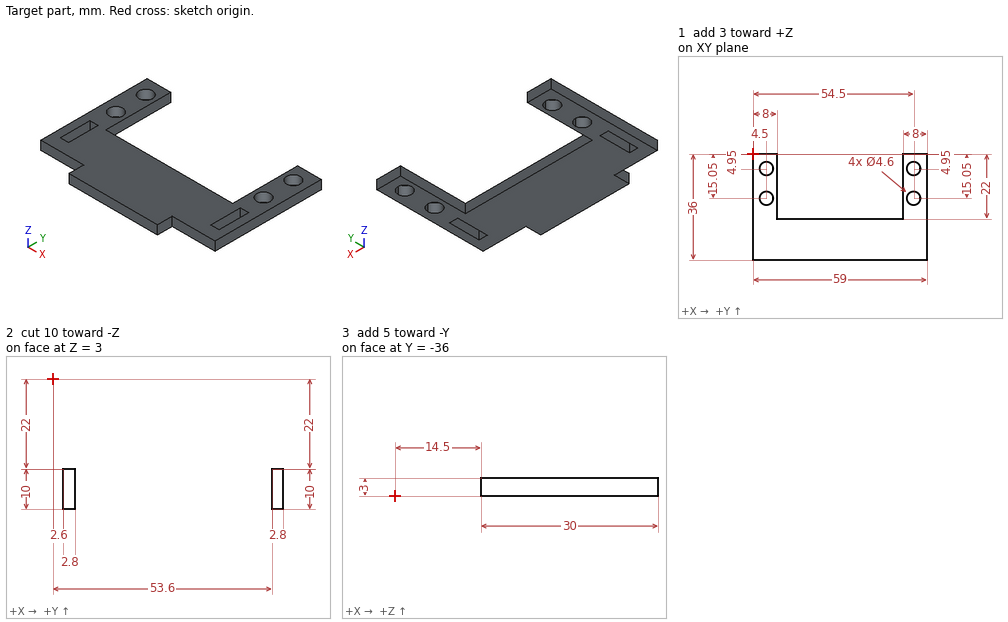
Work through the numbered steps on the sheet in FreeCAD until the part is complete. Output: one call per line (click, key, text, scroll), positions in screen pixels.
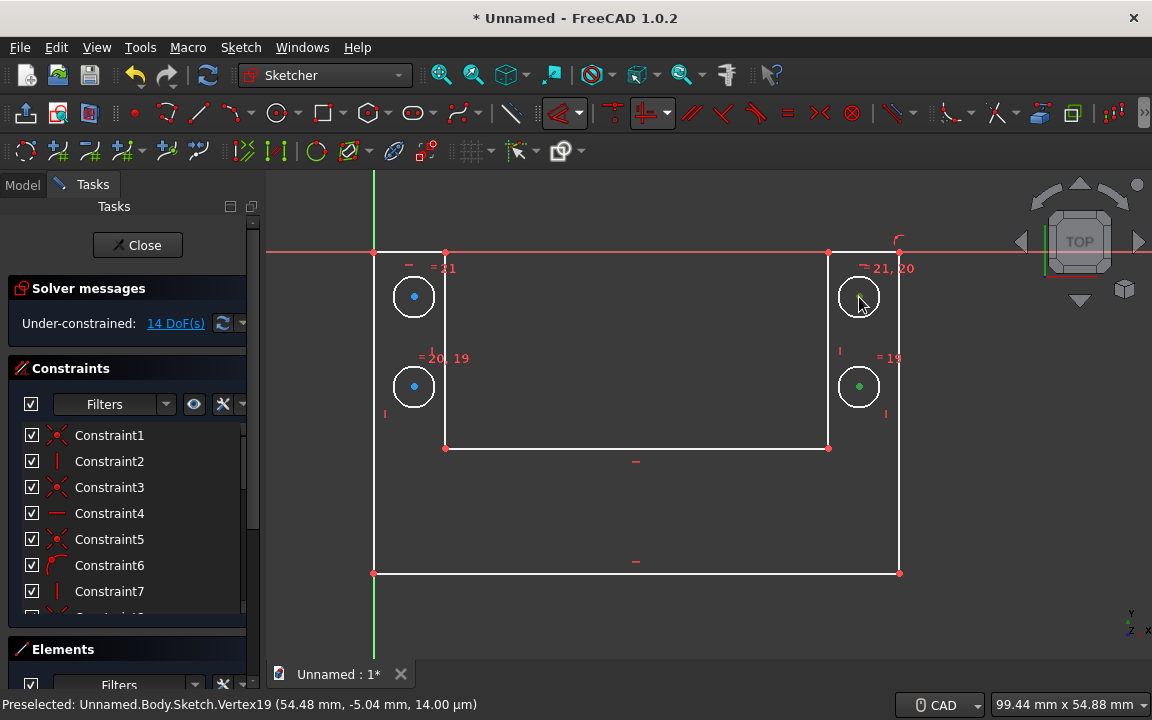
click(670, 114)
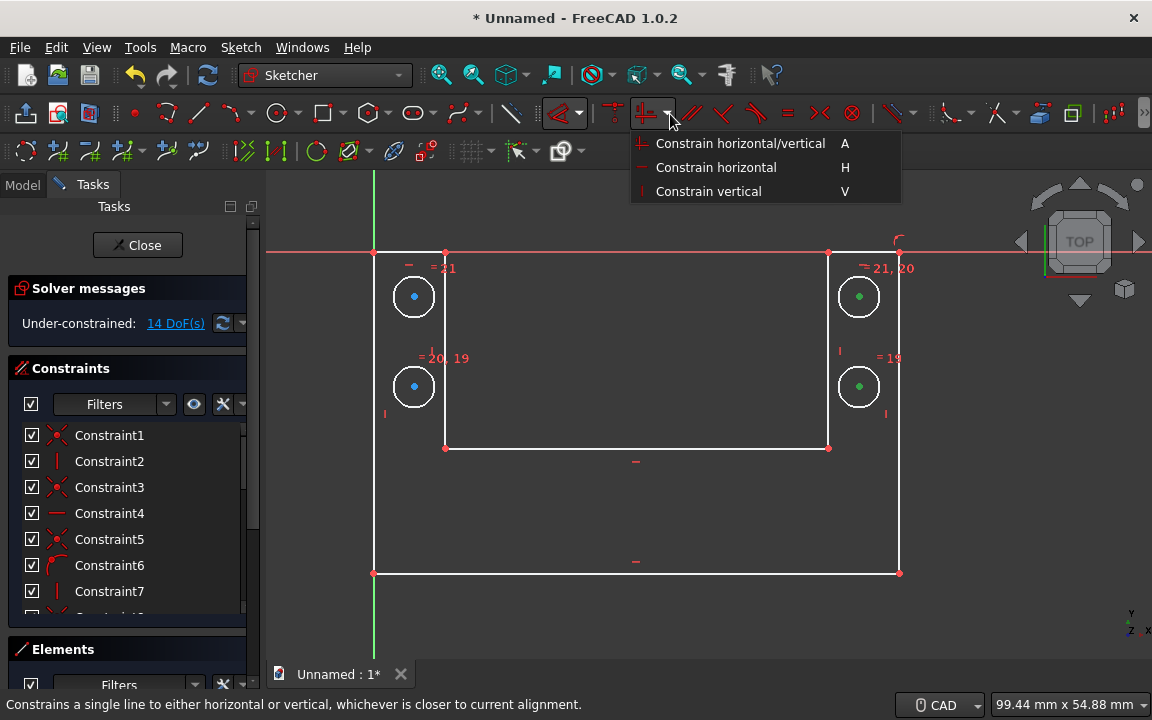
click(766, 191)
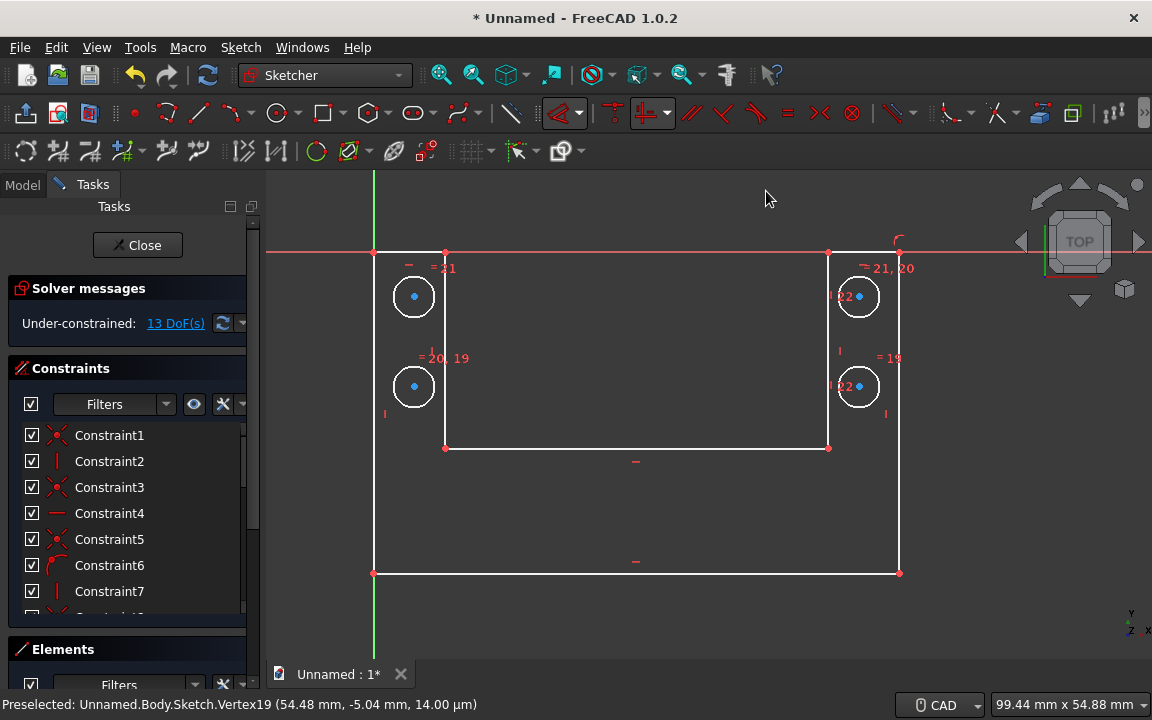
click(414, 387)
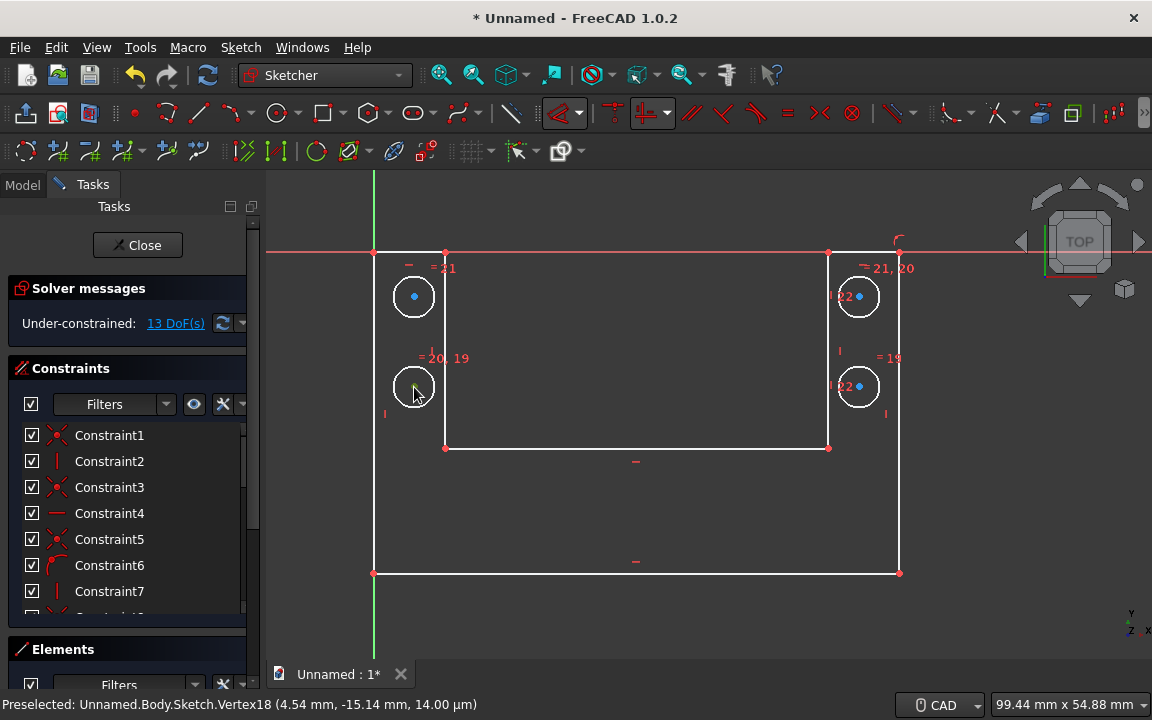
click(414, 297)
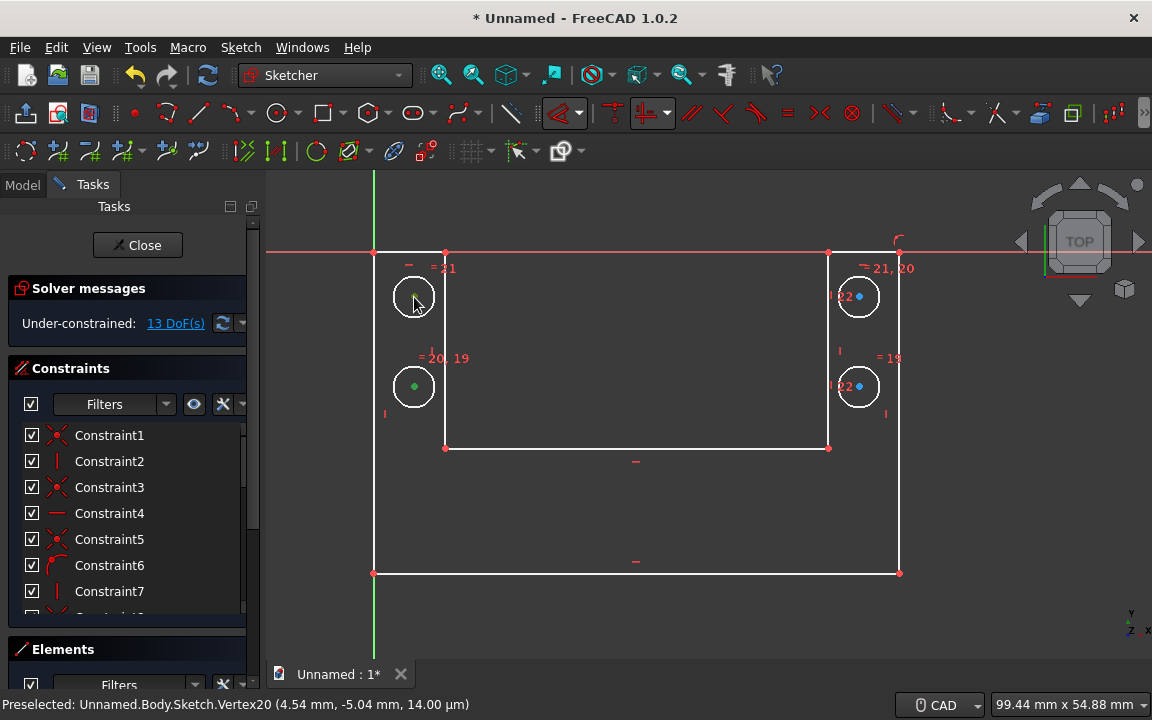
key(v)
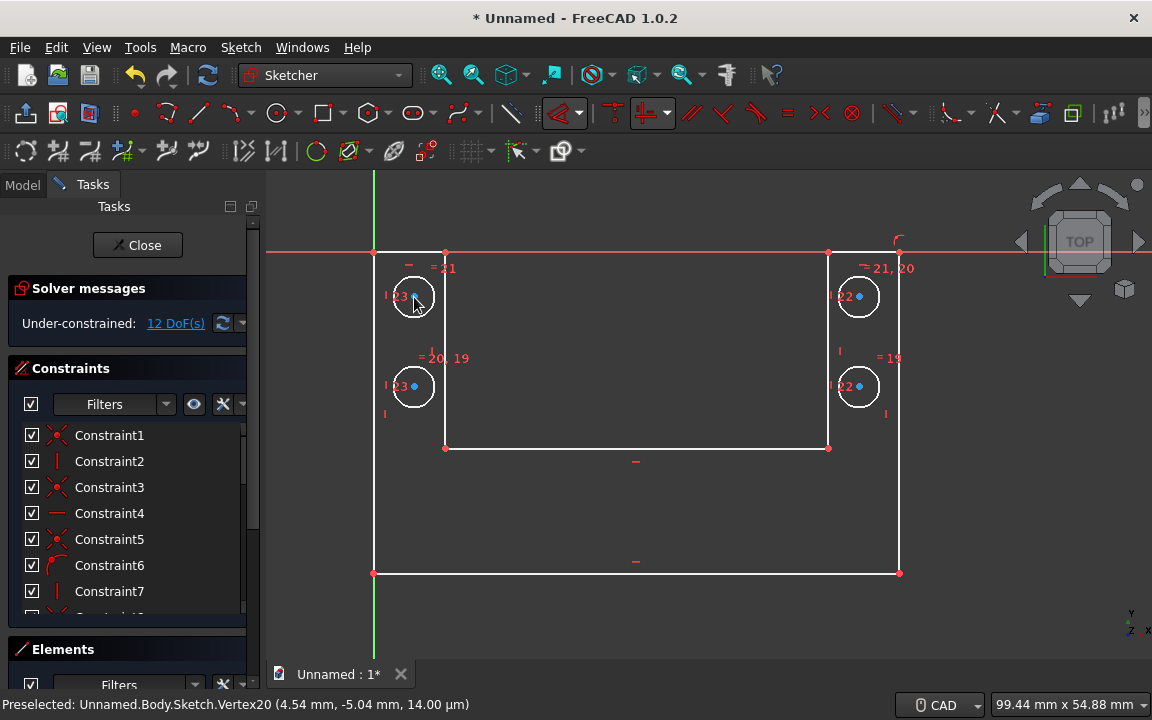
key(d)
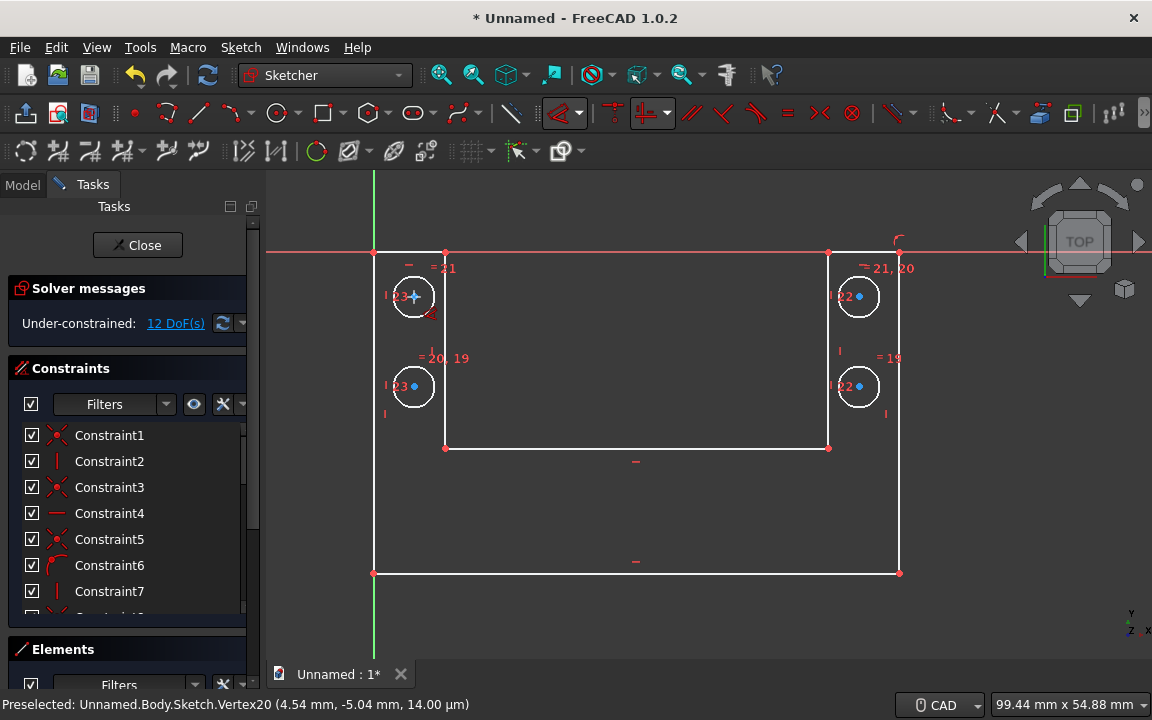
click(873, 372)
click(872, 336)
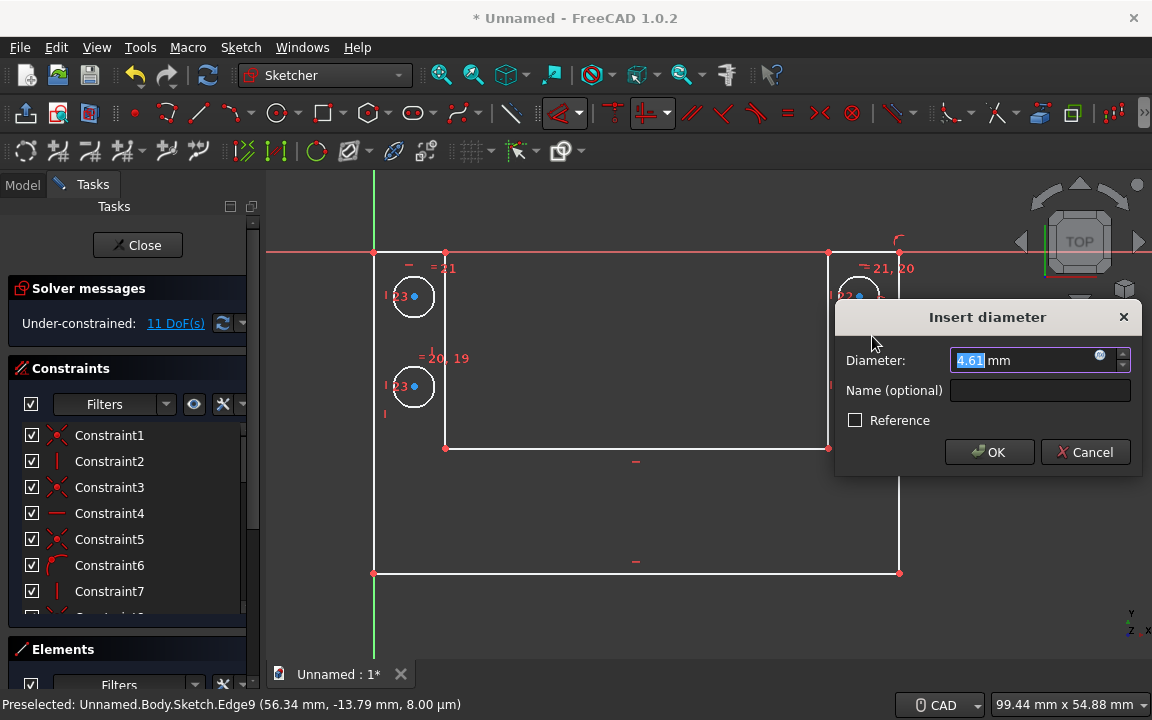
text(4.6)
key(Return)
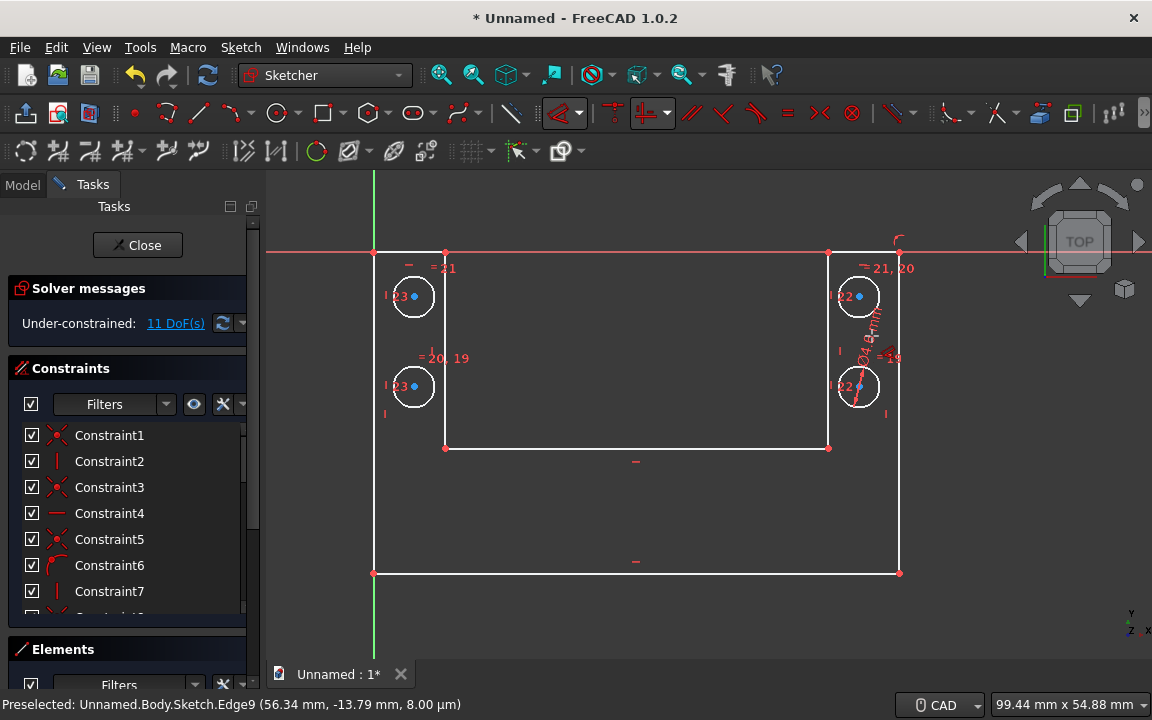
click(878, 252)
click(863, 218)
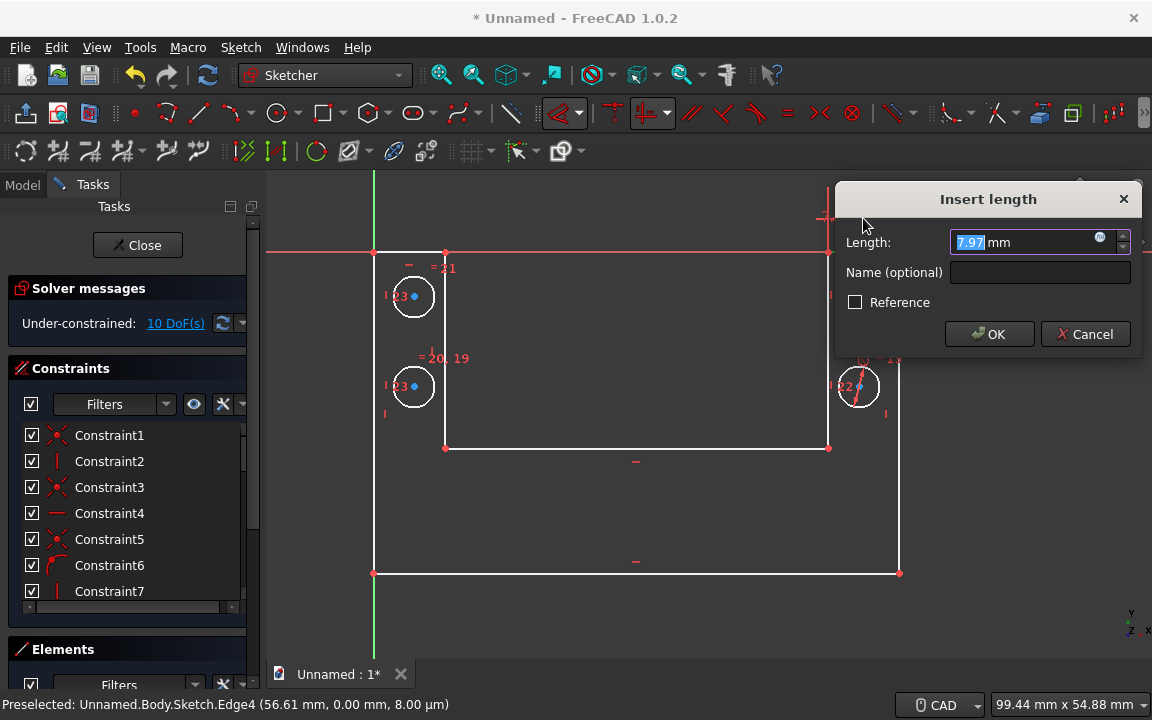
text(8)
key(Return)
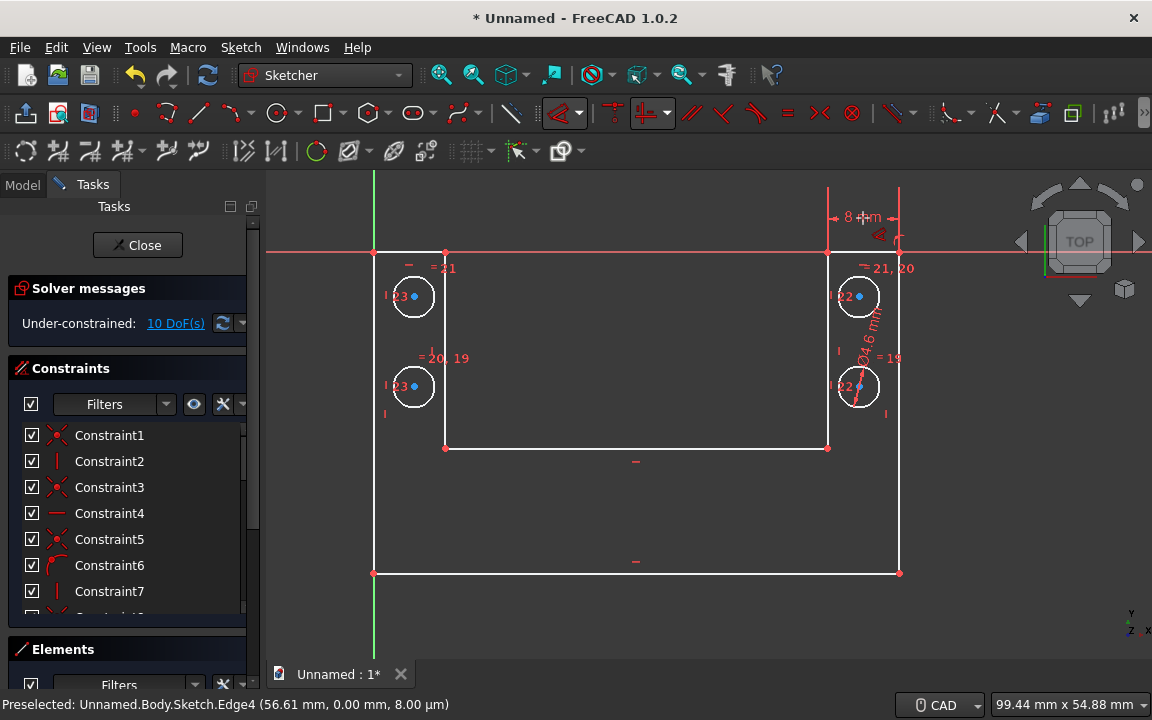
click(424, 252)
click(409, 218)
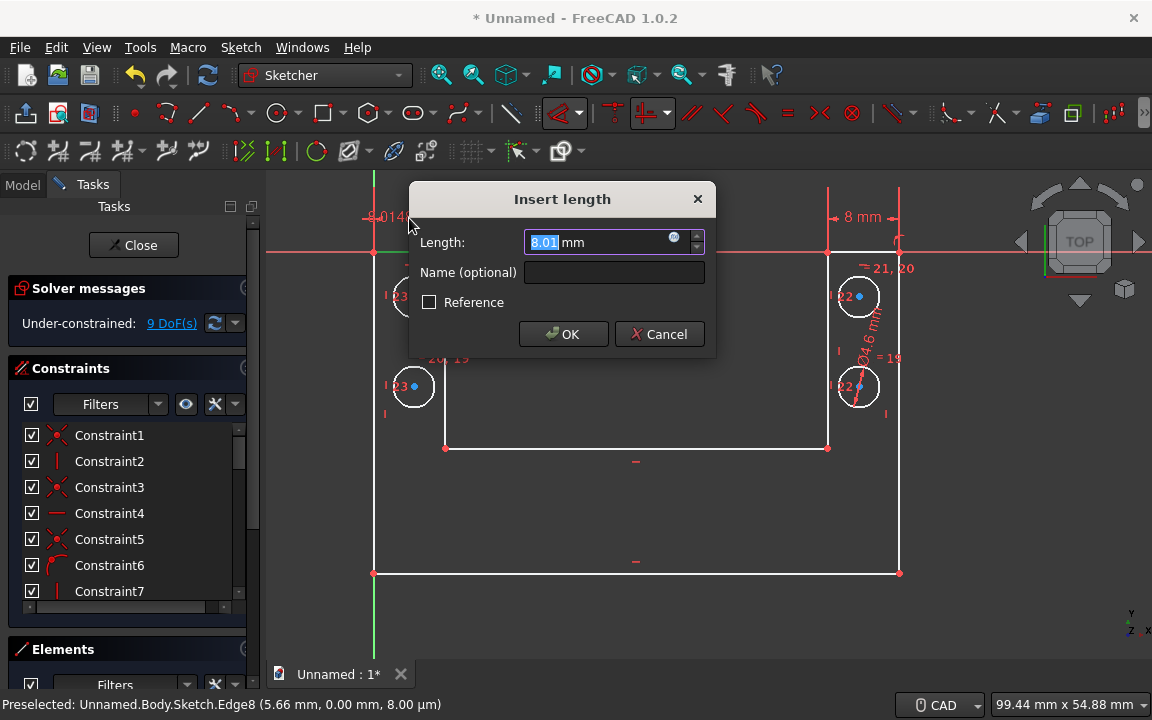
text(8)
key(Return)